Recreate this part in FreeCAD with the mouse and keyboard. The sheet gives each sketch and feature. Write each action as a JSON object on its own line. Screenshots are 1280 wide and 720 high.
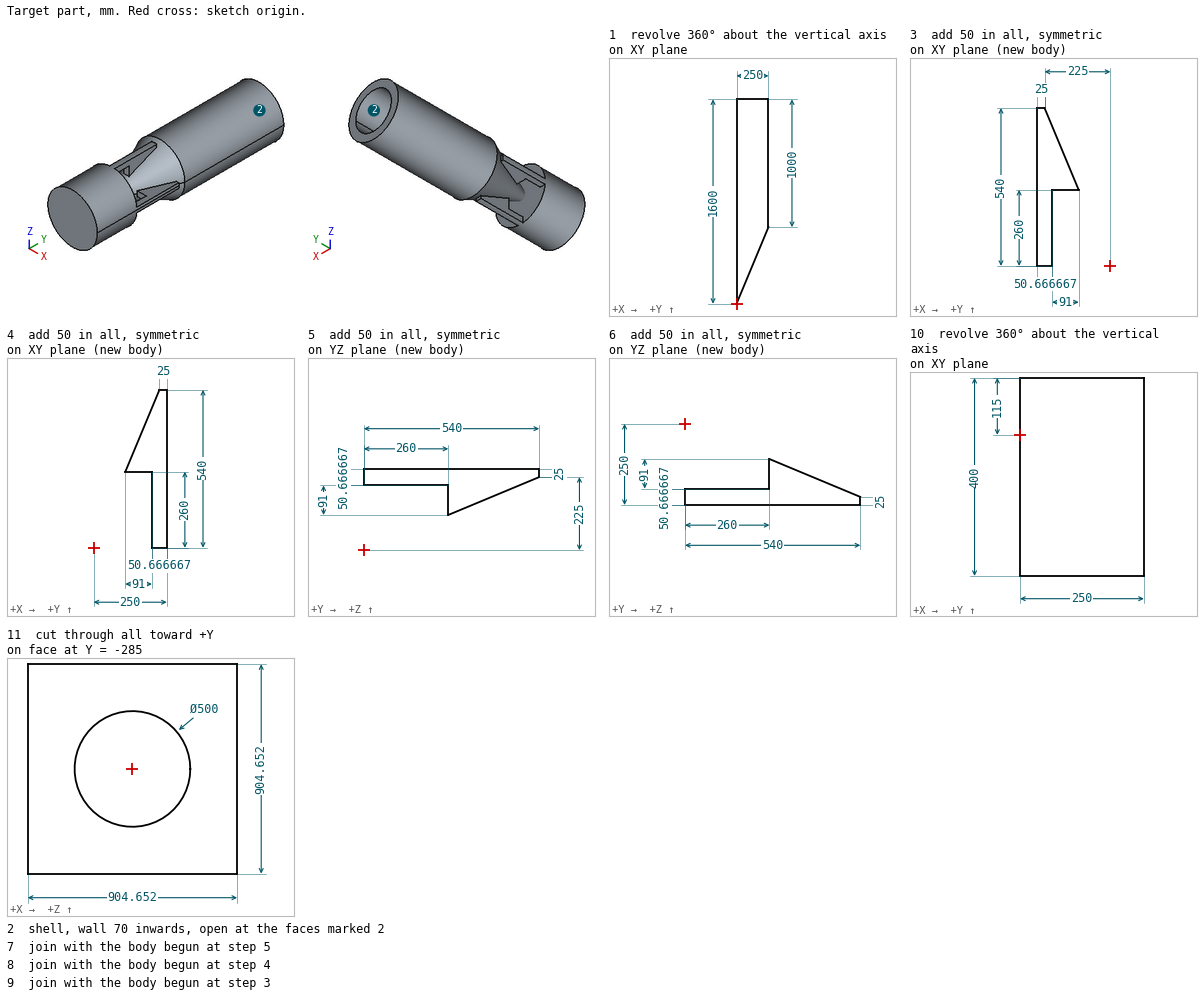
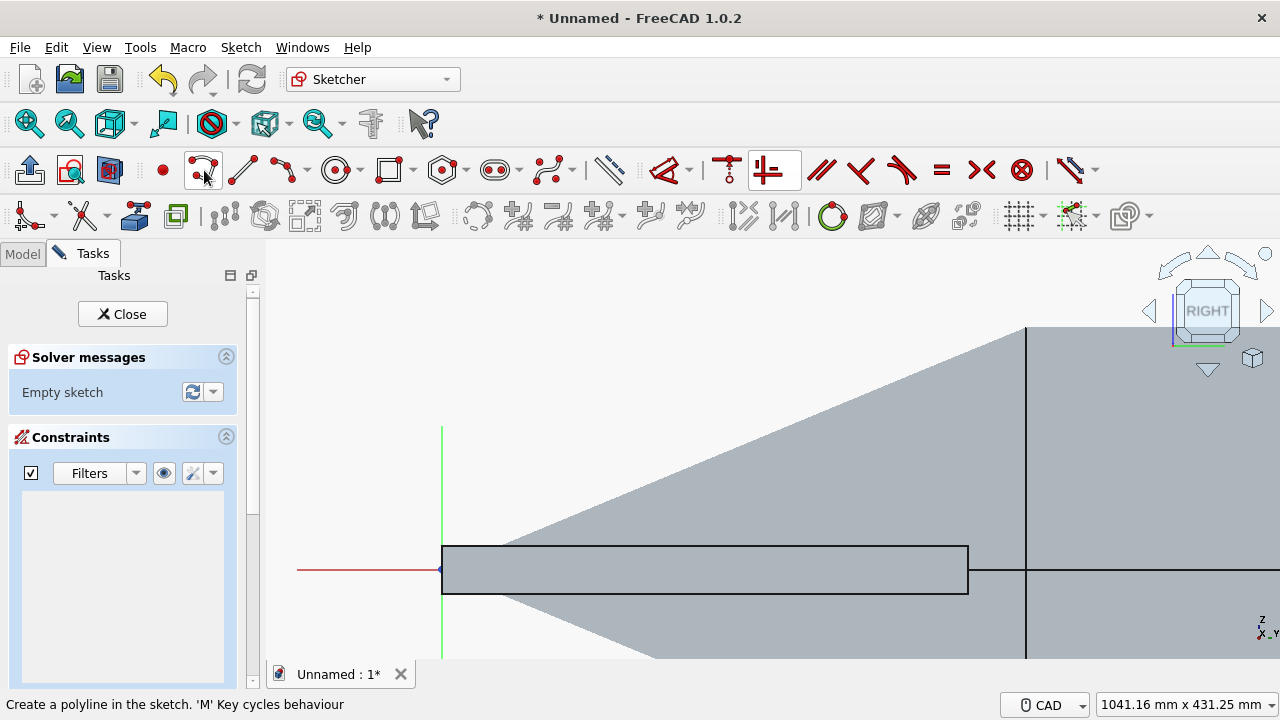
{"action": "left_click", "coordinate": [442, 376]}
{"action": "left_click", "coordinate": [695, 376]}
{"action": "left_click", "coordinate": [695, 464]}
{"action": "left_click", "coordinate": [968, 351]}
{"action": "left_click", "coordinate": [968, 326]}
{"action": "left_click", "coordinate": [451, 326]}
{"action": "left_click", "coordinate": [442, 377]}
{"action": "key", "text": "Escape"}
{"action": "key", "text": "Escape"}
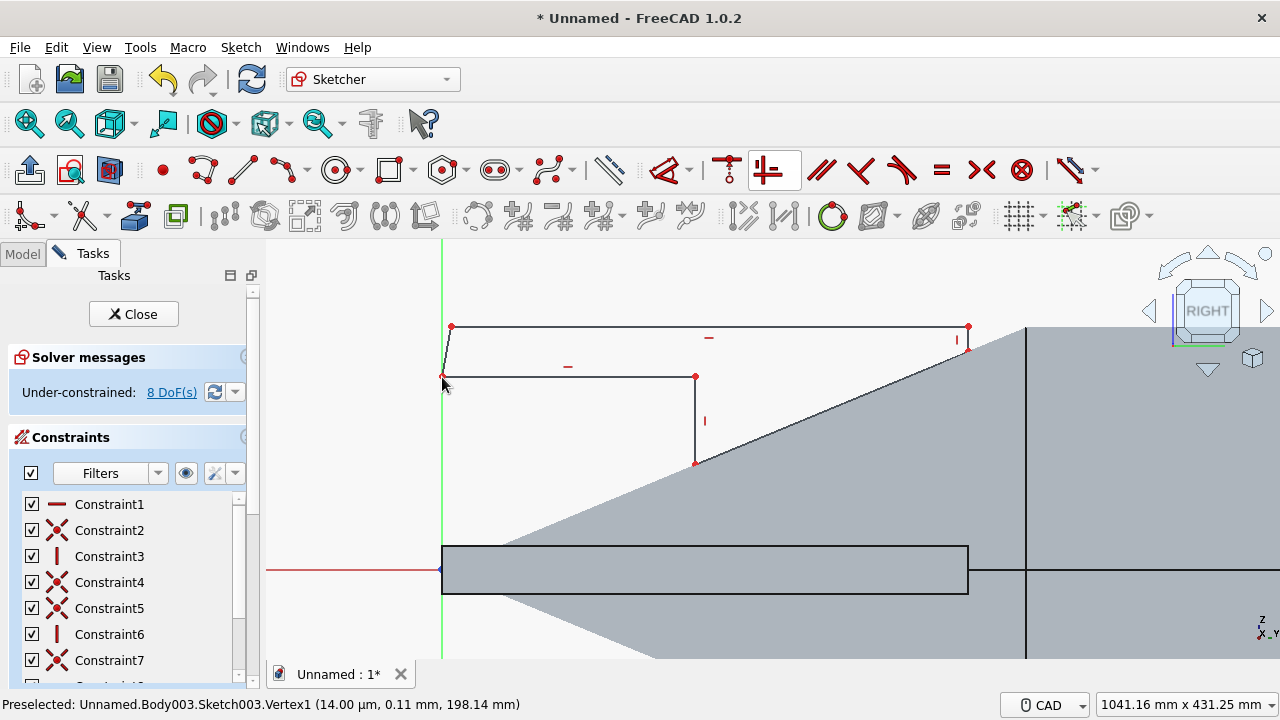
{"action": "left_click", "coordinate": [445, 362]}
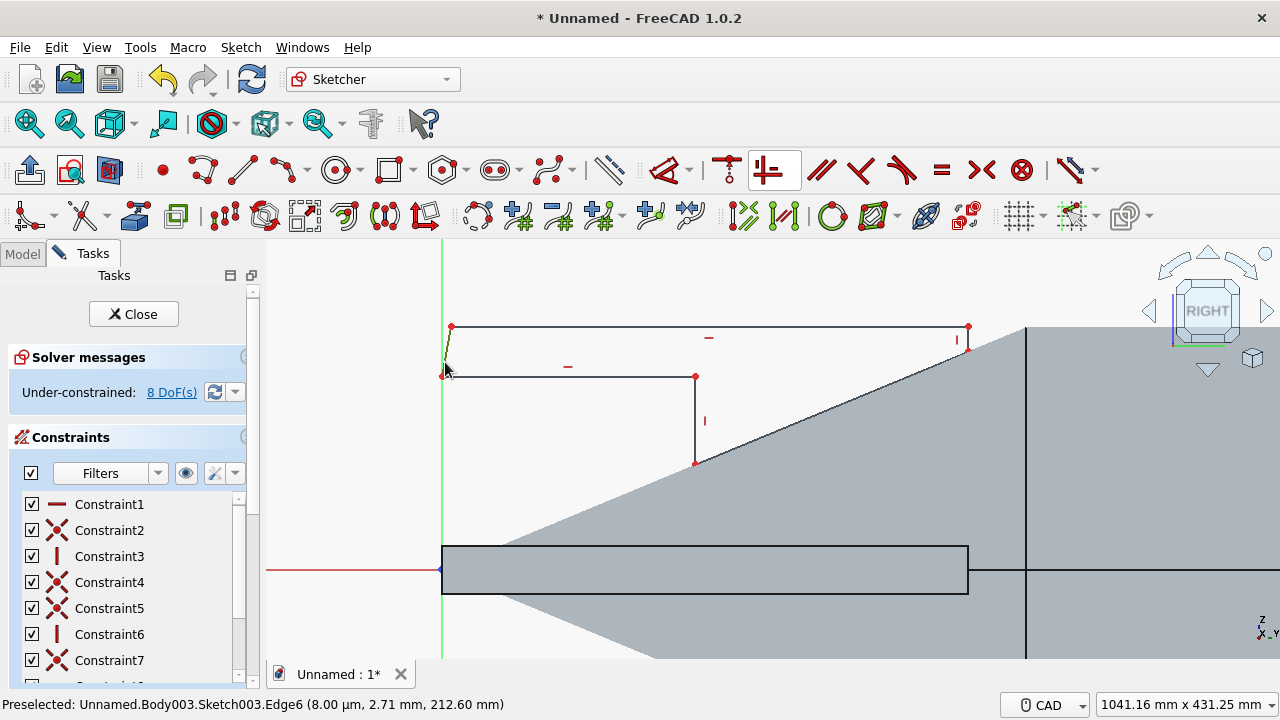
{"action": "key", "text": "v"}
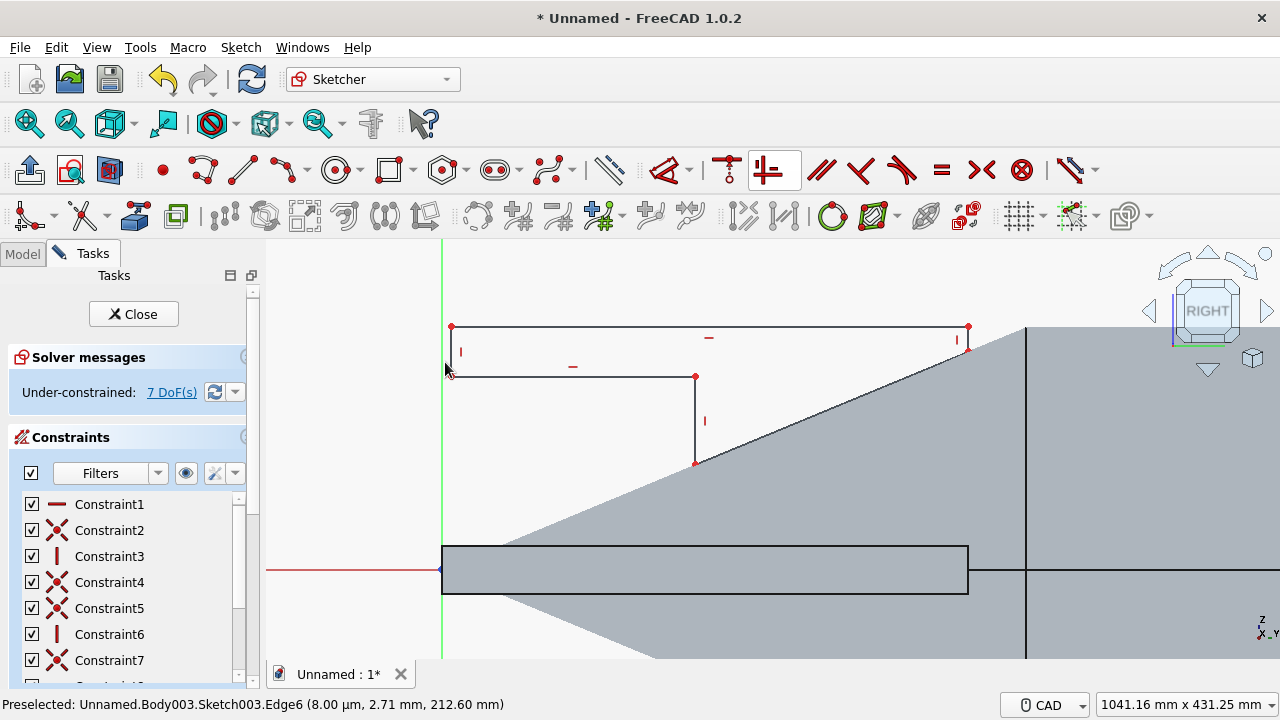
{"action": "left_click", "coordinate": [451, 377]}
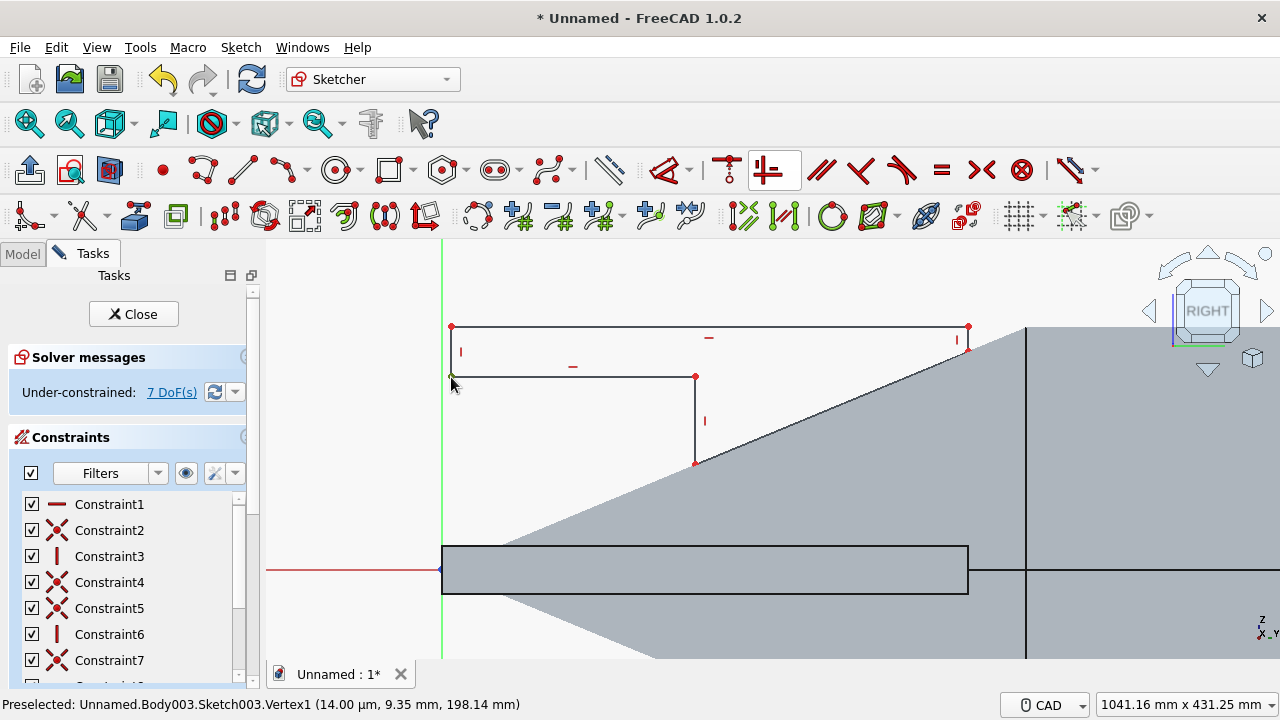
{"action": "left_click", "coordinate": [442, 605]}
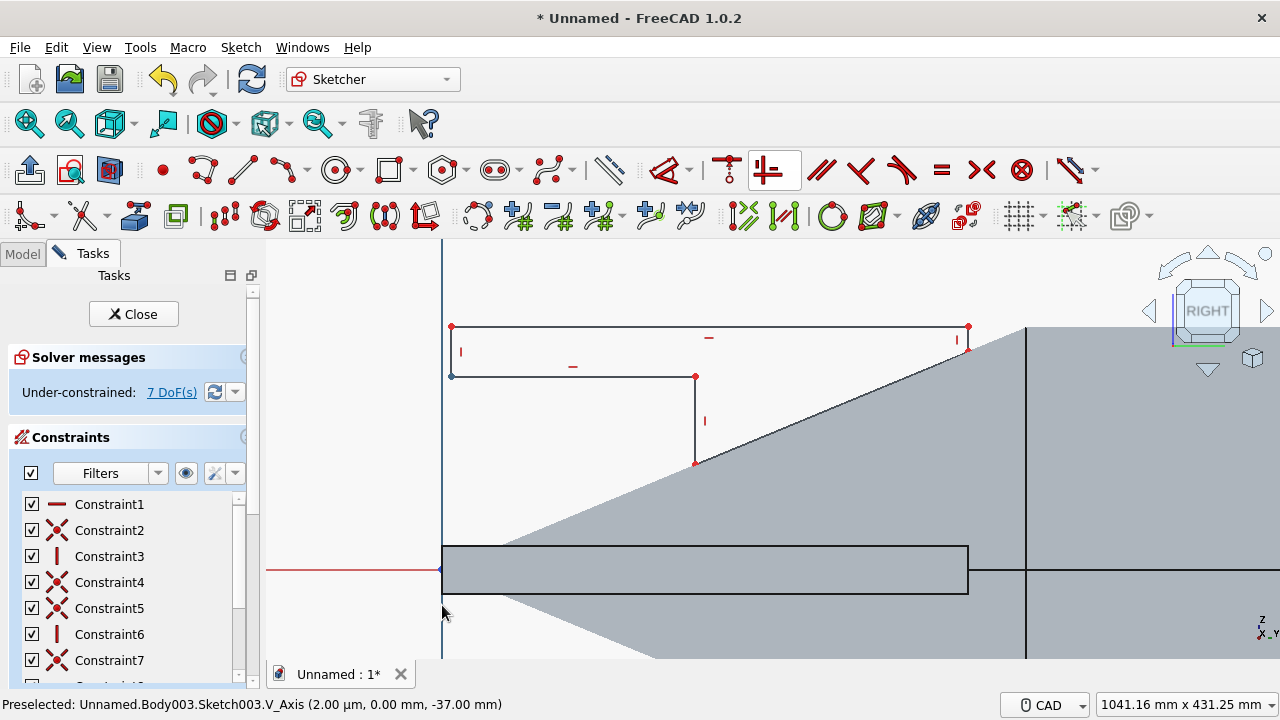
{"action": "left_click", "coordinate": [728, 170]}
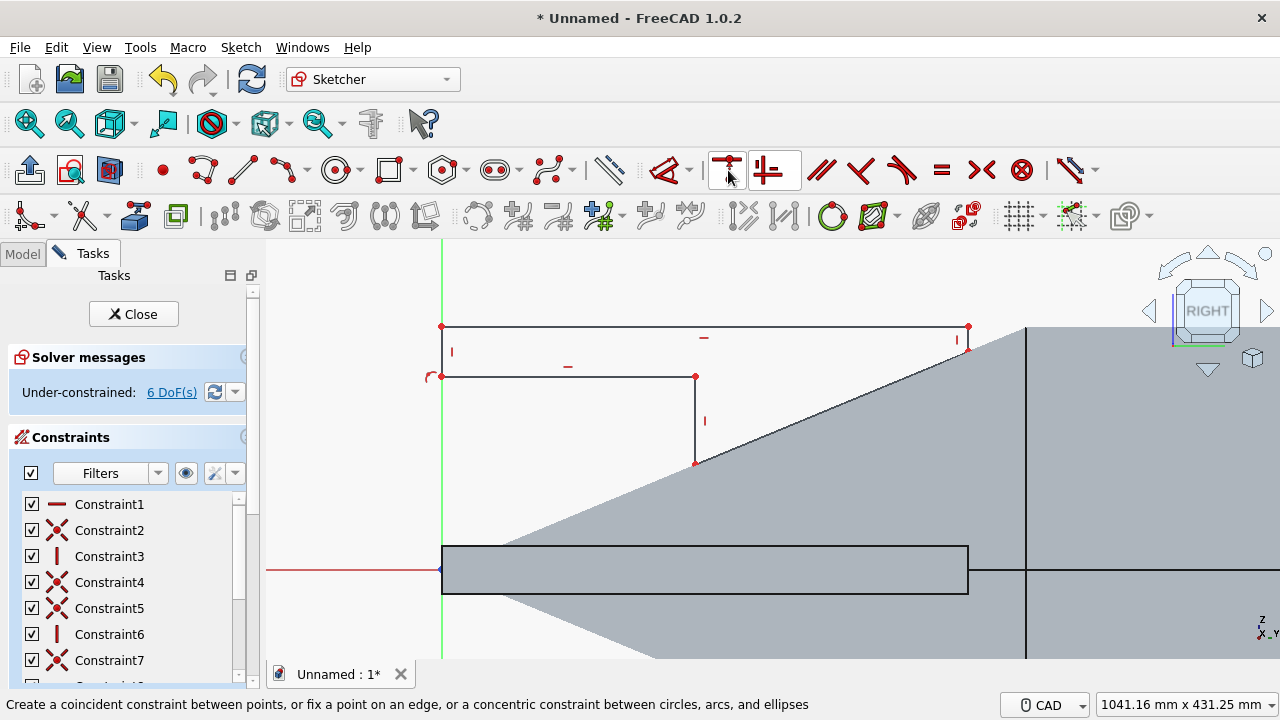
{"action": "left_click", "coordinate": [664, 170]}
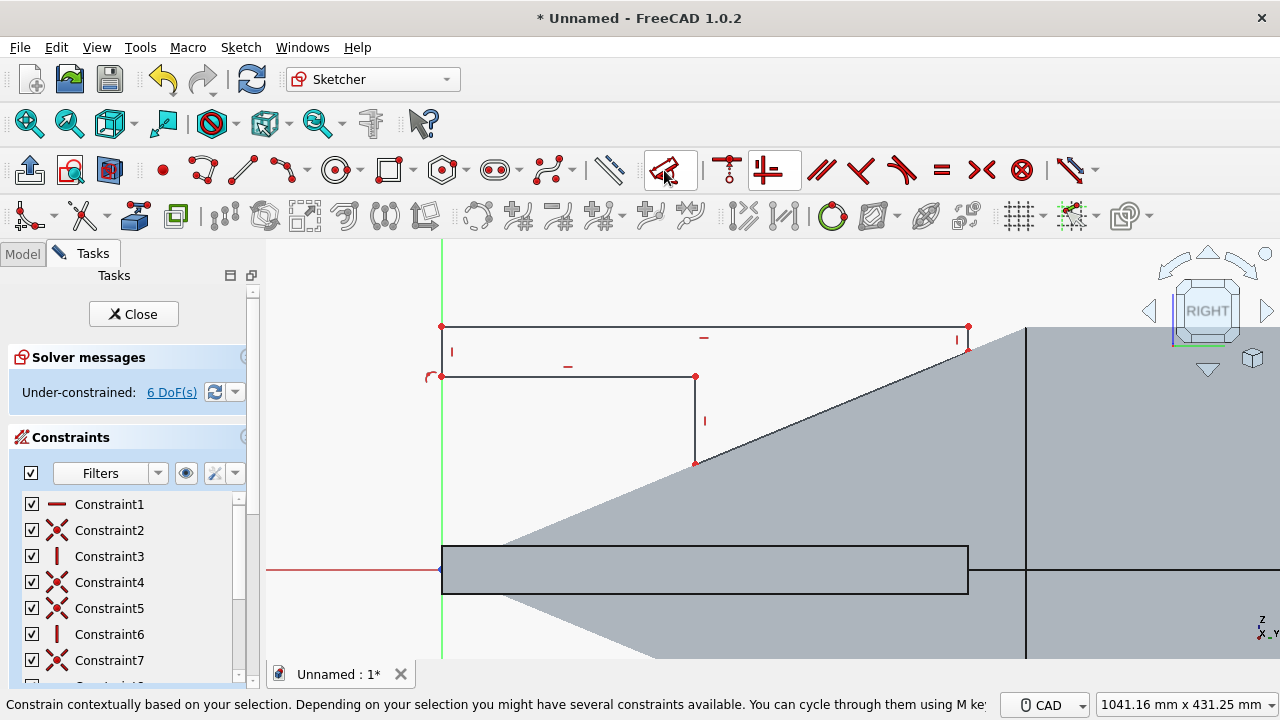
{"action": "left_click", "coordinate": [695, 403]}
{"action": "left_click", "coordinate": [661, 421]}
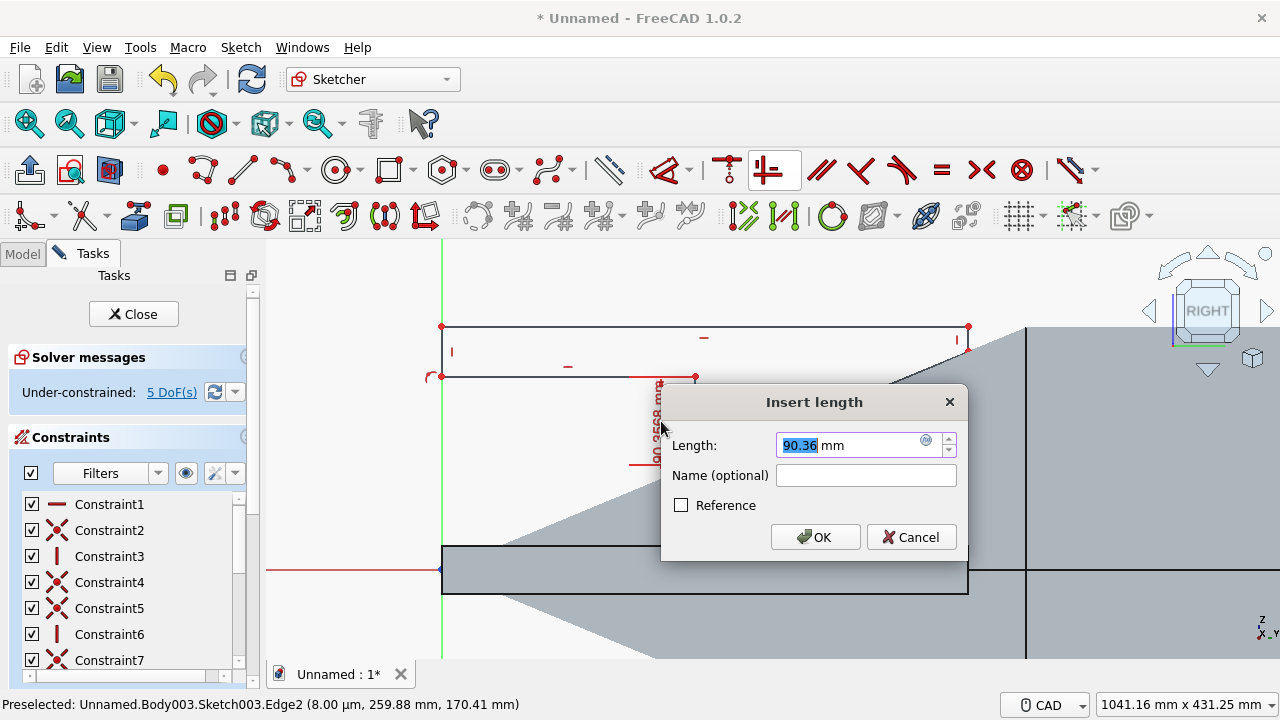
{"action": "type", "text": "91"}
{"action": "key", "text": "Return"}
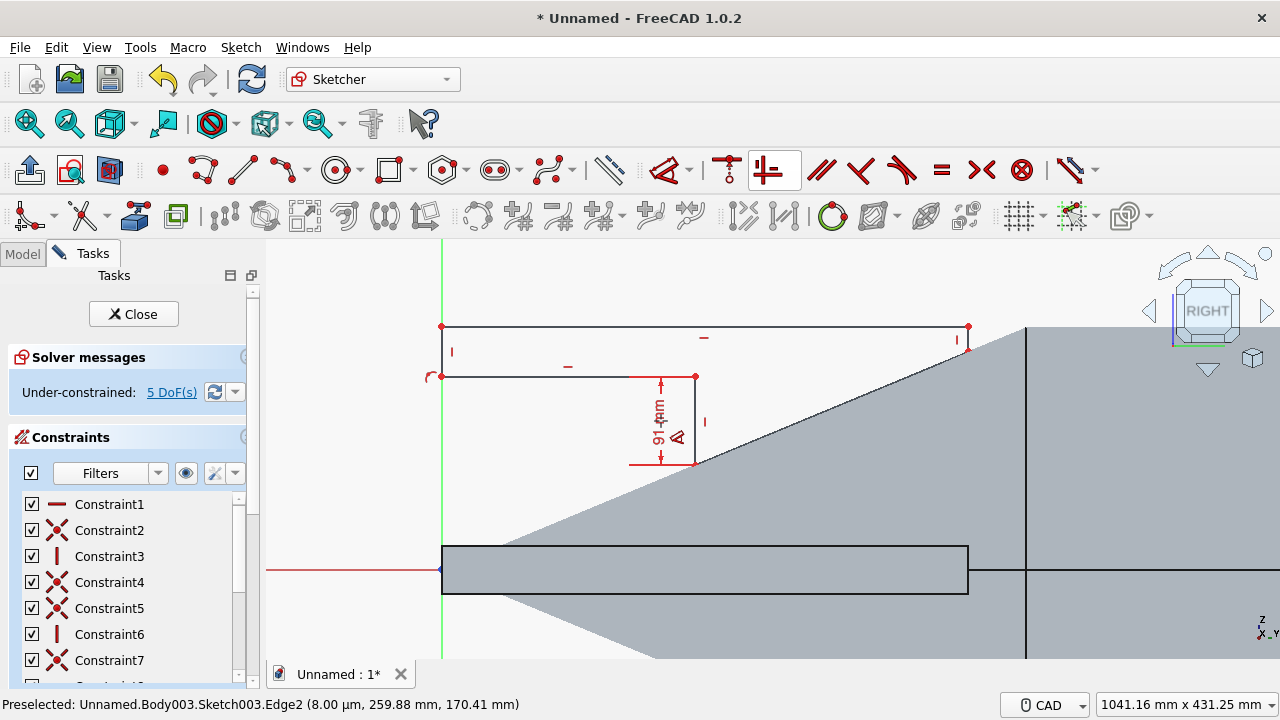
{"action": "scroll", "coordinate": [968, 342], "scroll_direction": "up", "scroll_amount": 3}